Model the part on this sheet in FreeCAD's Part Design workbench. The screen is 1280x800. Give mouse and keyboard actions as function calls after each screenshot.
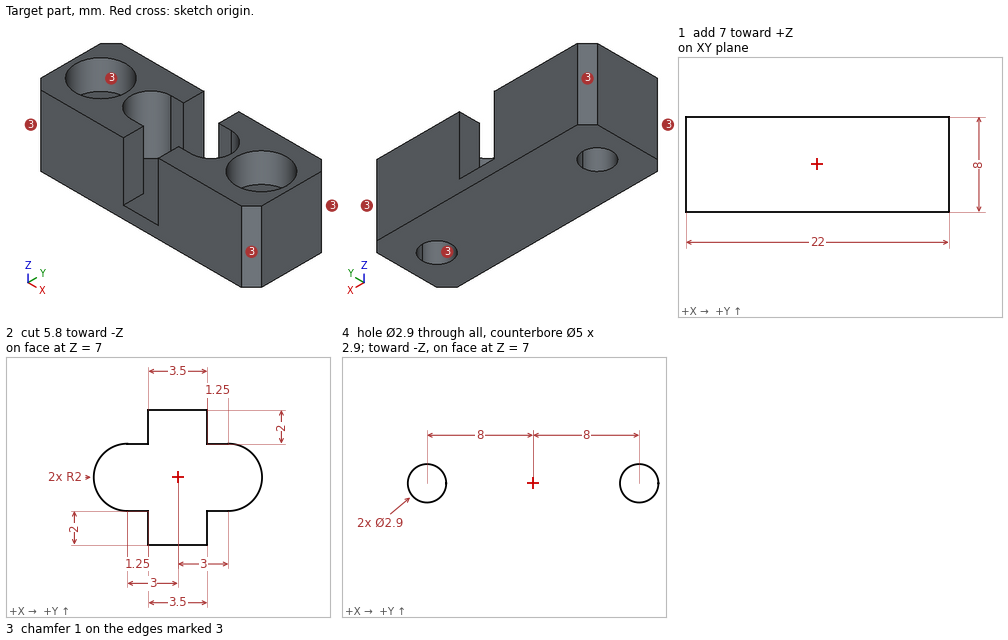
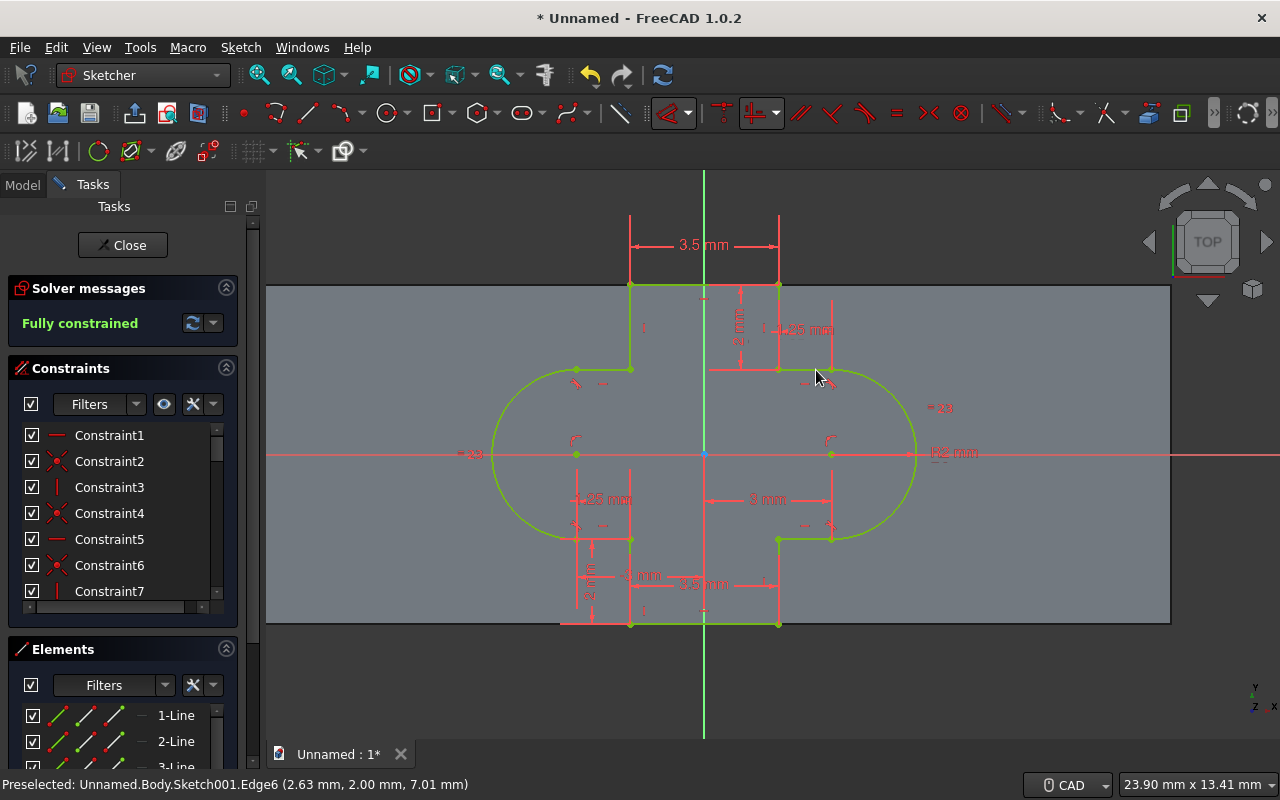
click(123, 245)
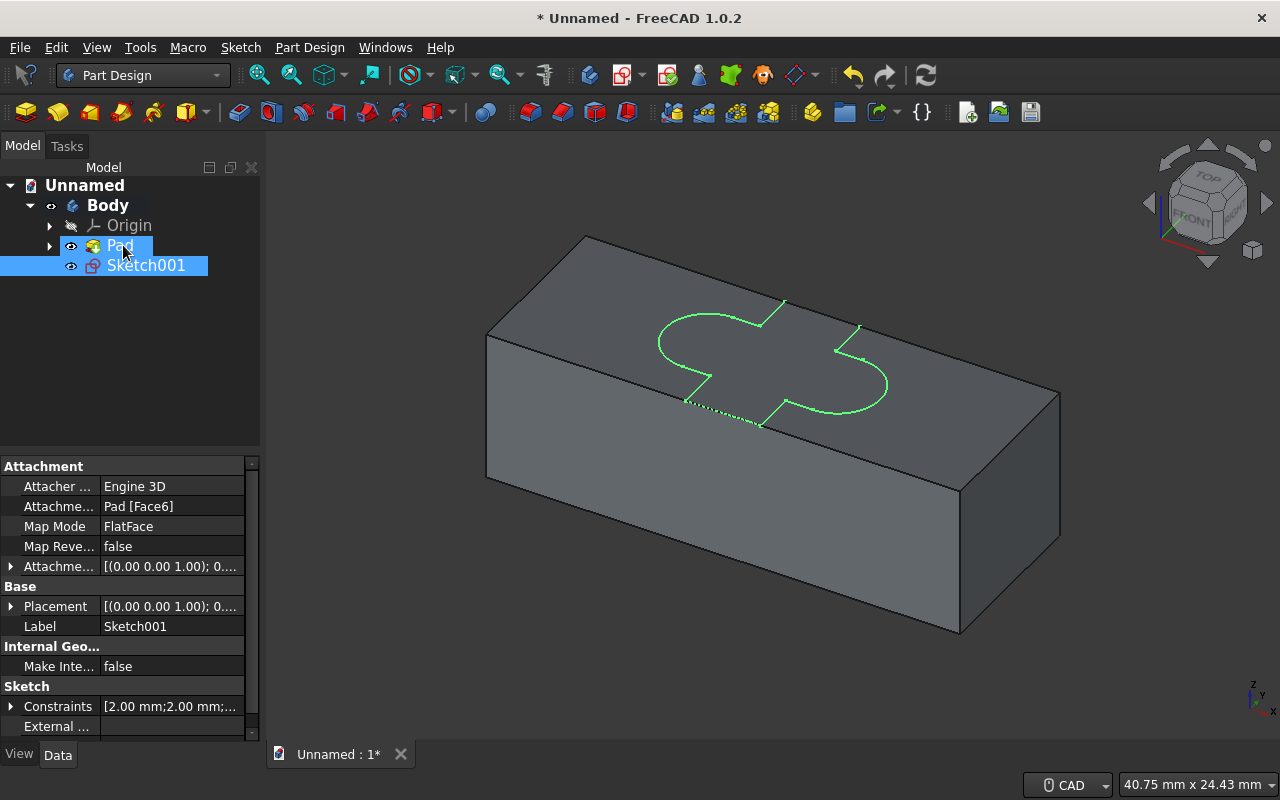
click(240, 112)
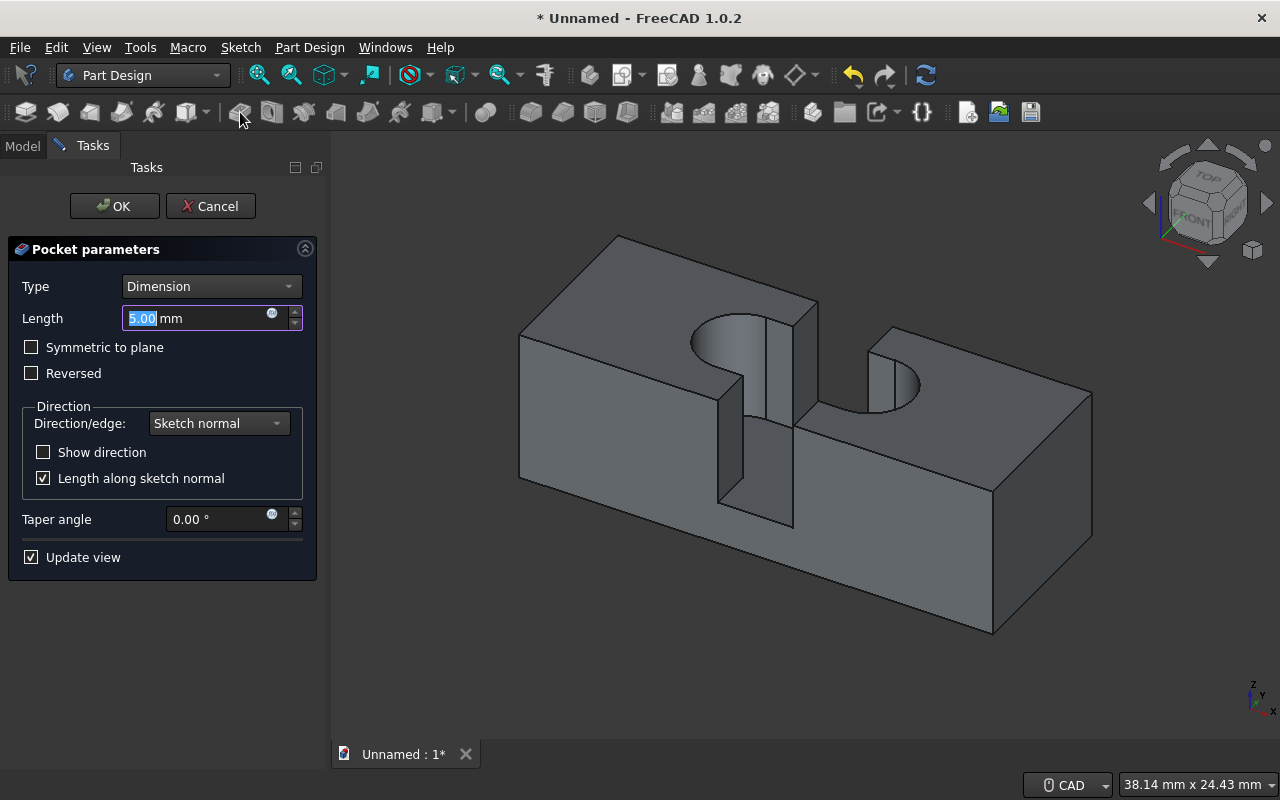
text(5.8)
key(Tab)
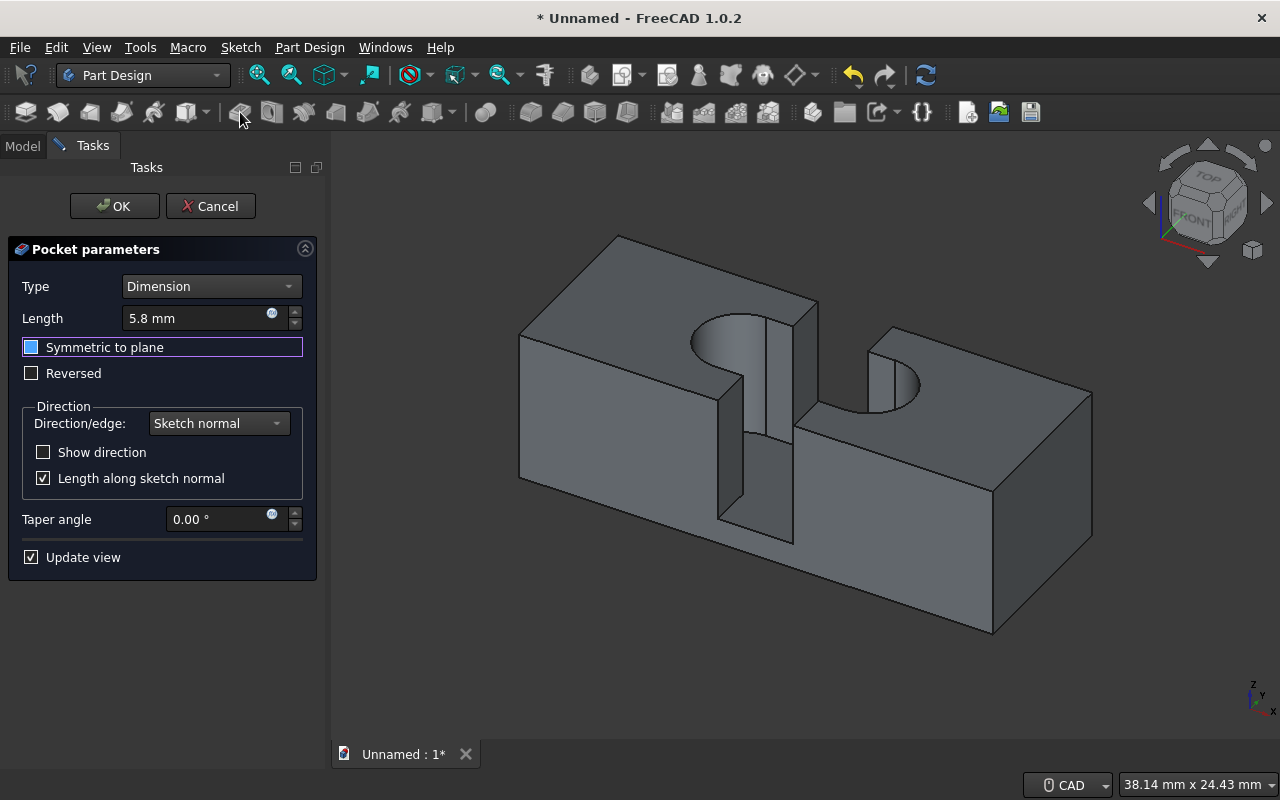
click(115, 206)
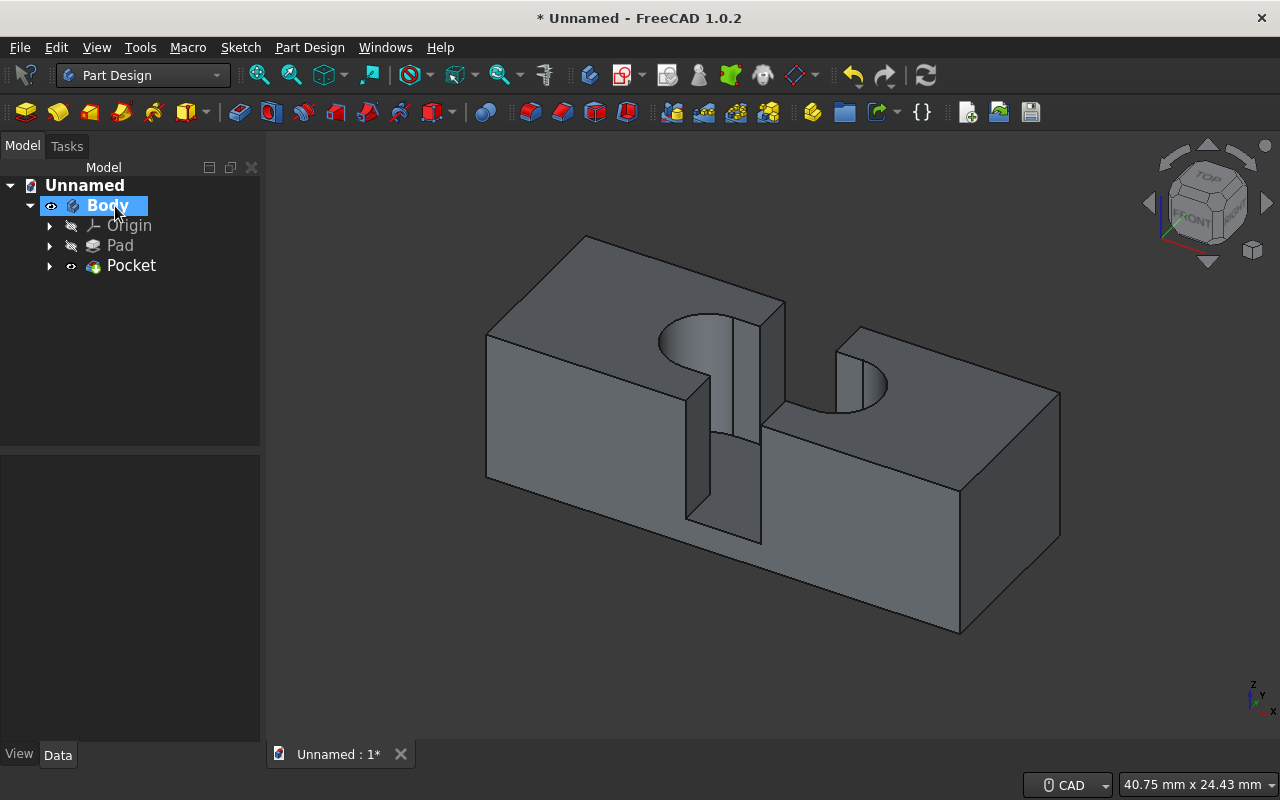
click(960, 562)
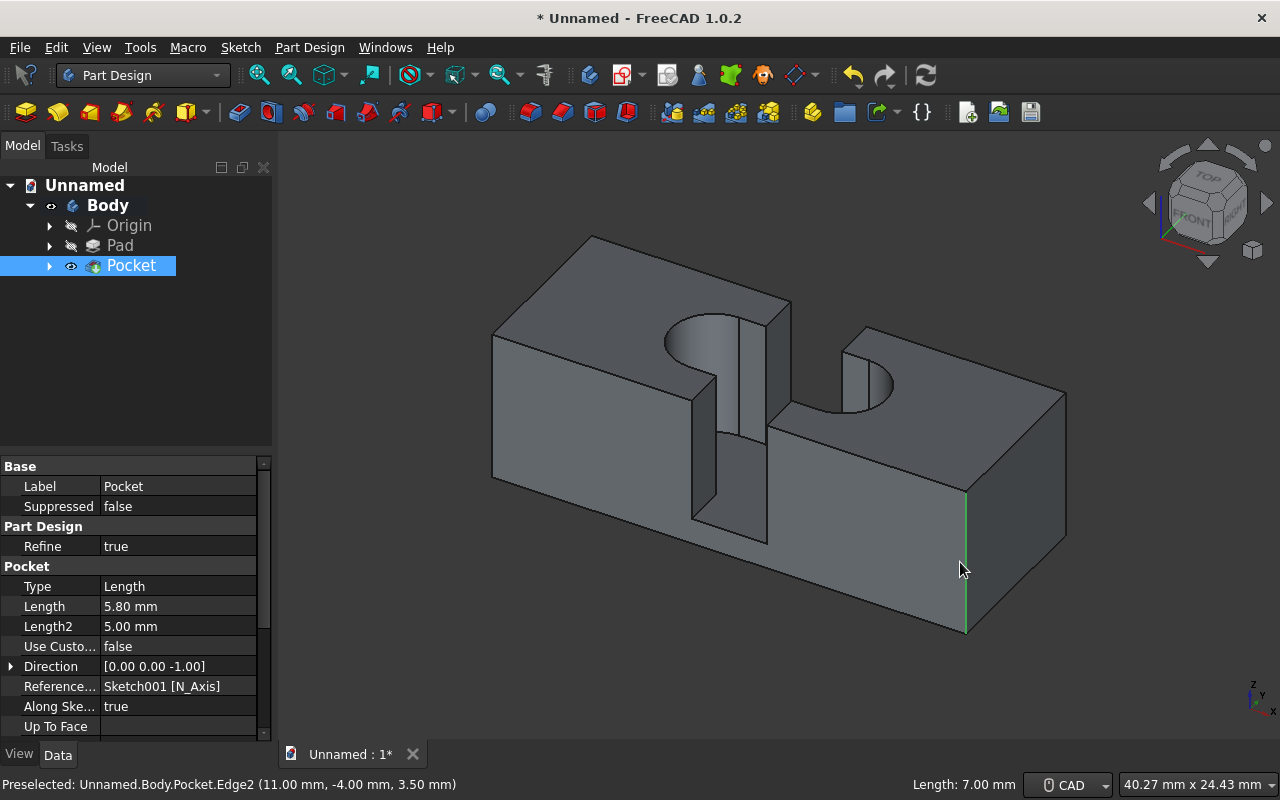
key(0)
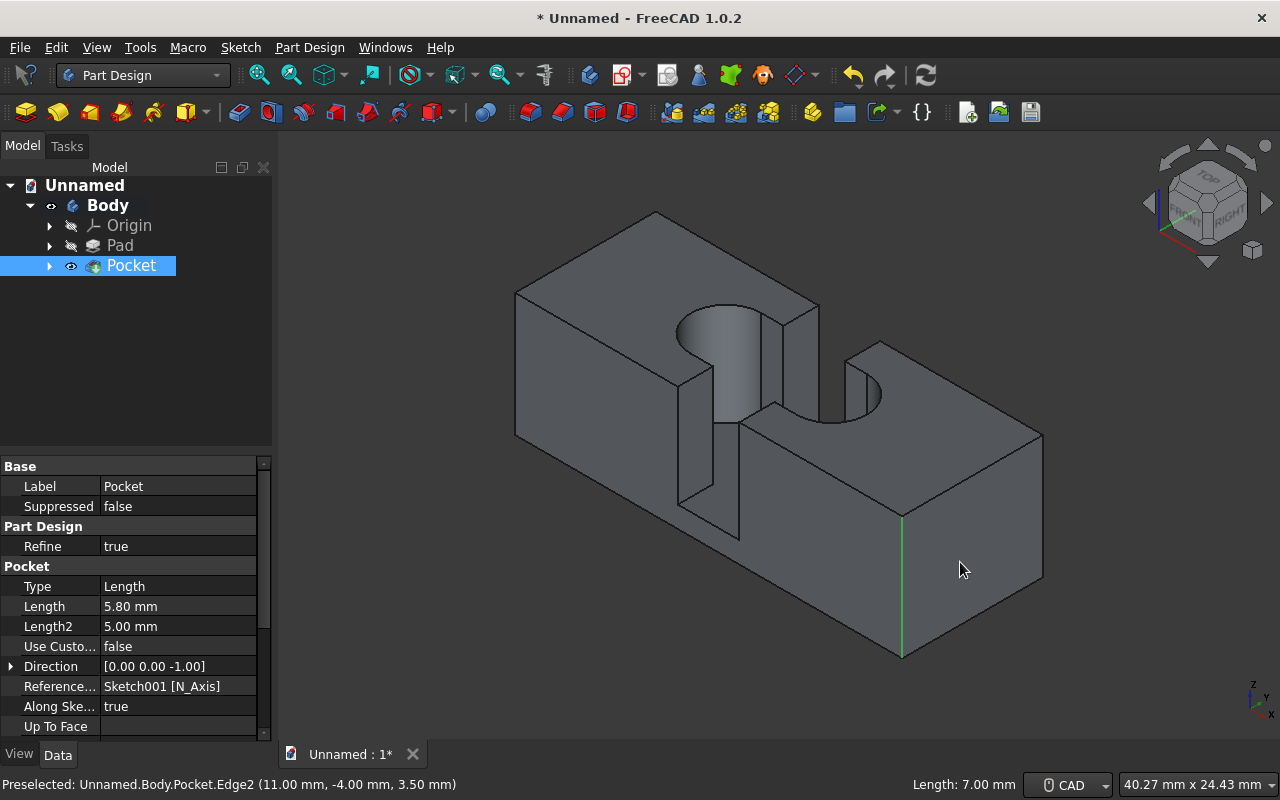
key(2)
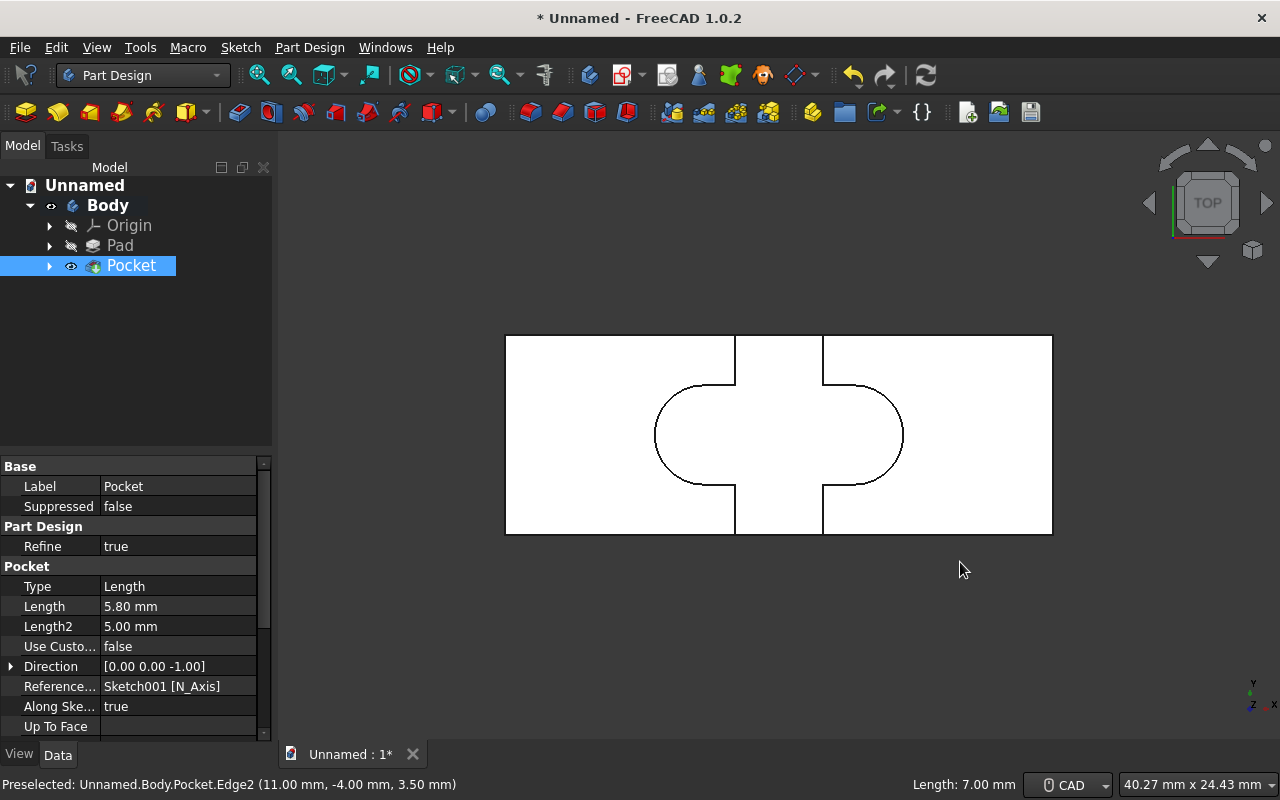
key(1)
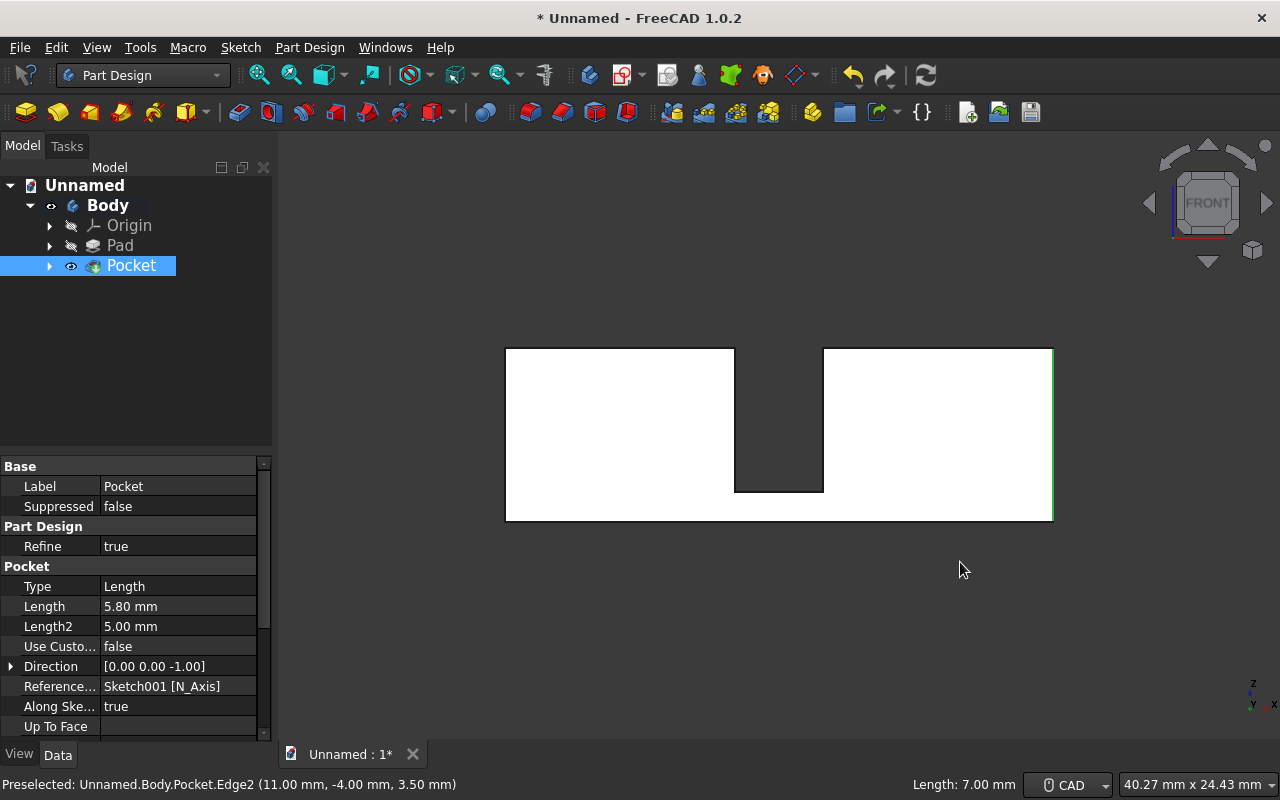
click(505, 434, ctrl)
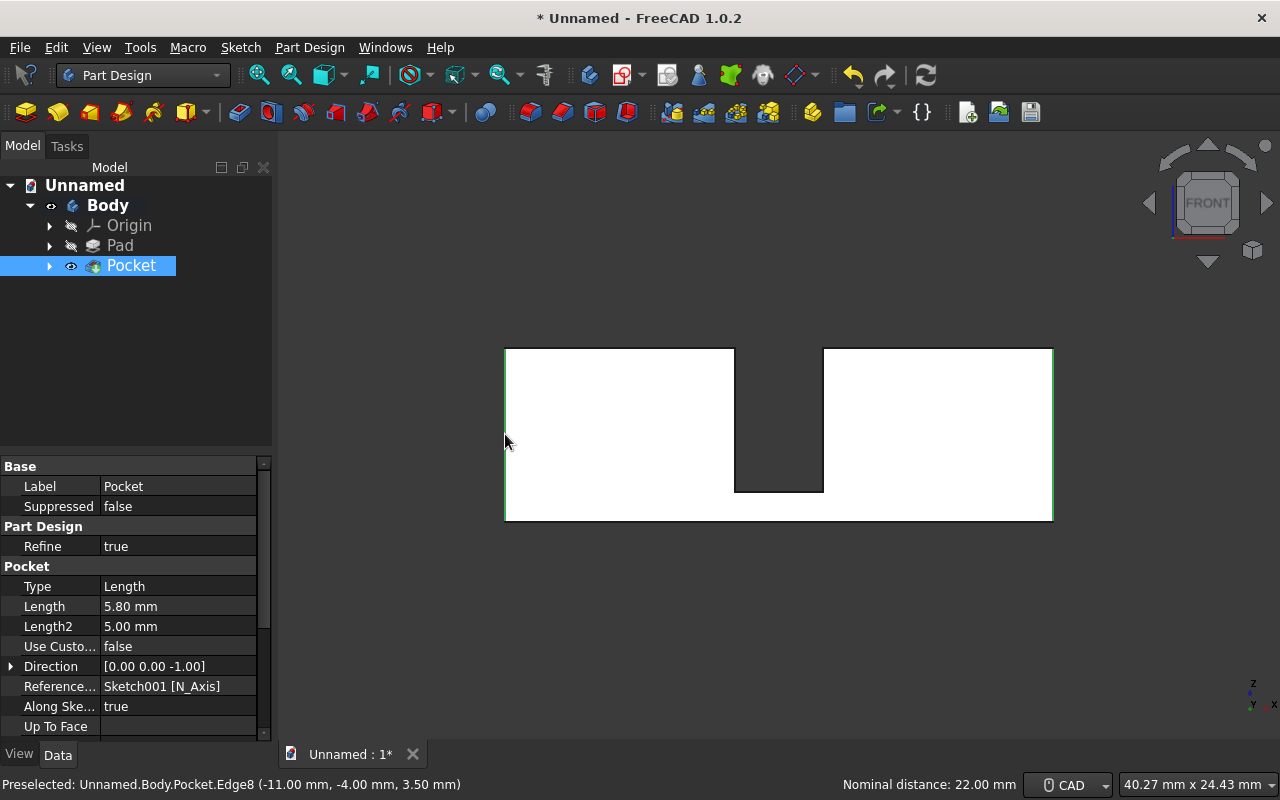
key(3)